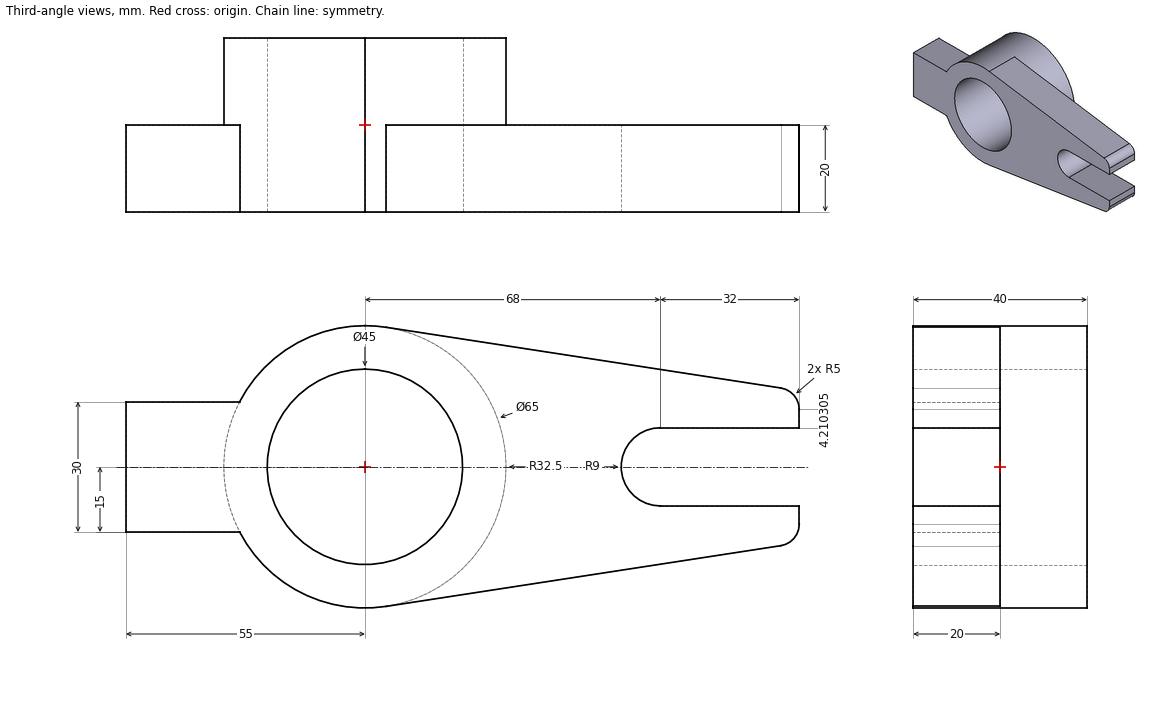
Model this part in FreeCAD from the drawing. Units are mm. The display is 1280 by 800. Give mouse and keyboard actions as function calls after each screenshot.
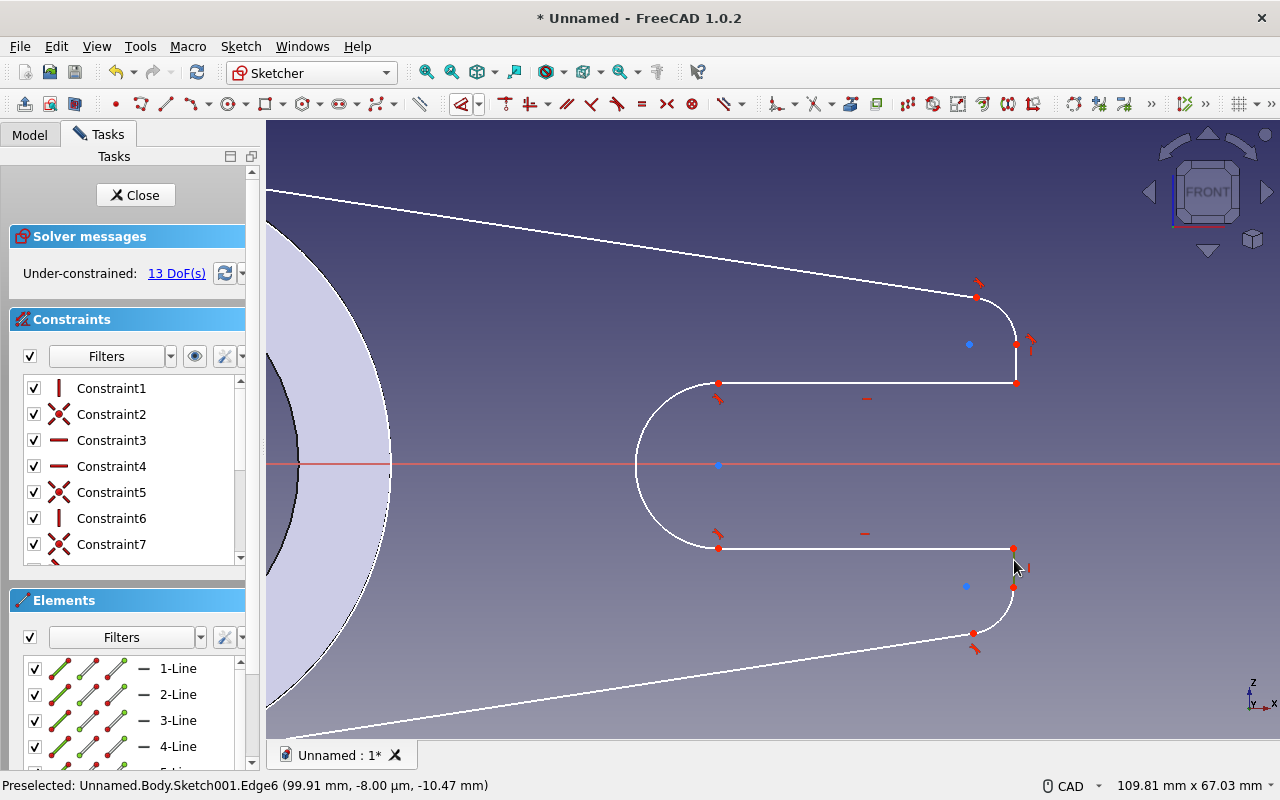
click(992, 627)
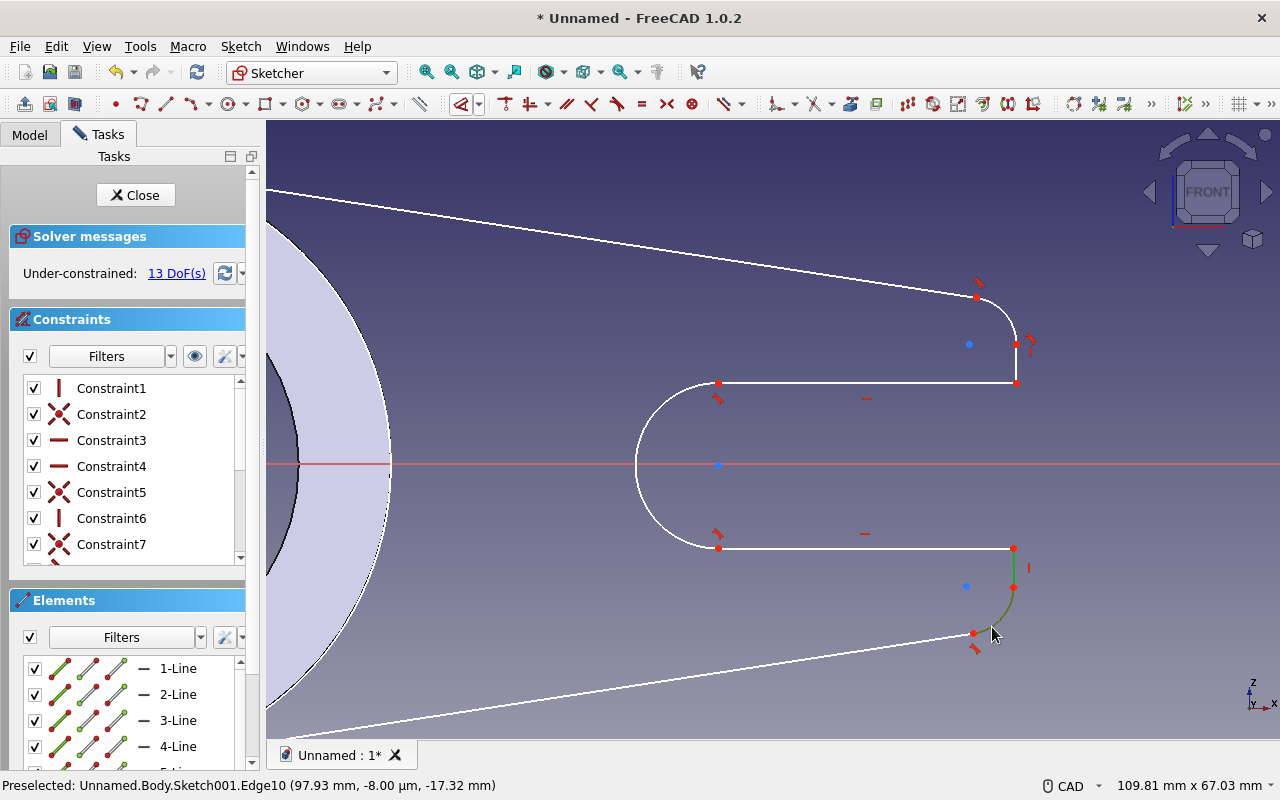
click(617, 104)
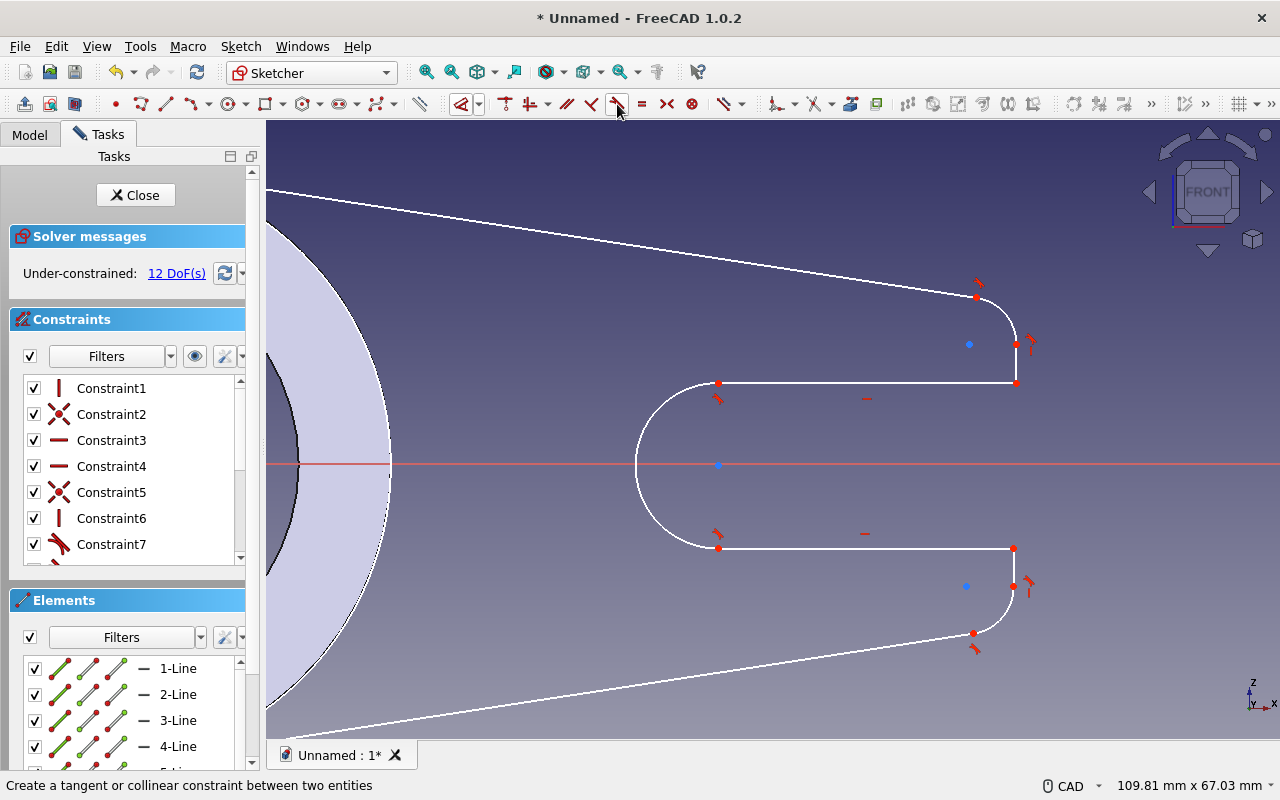
scroll(1013, 359, down, 2)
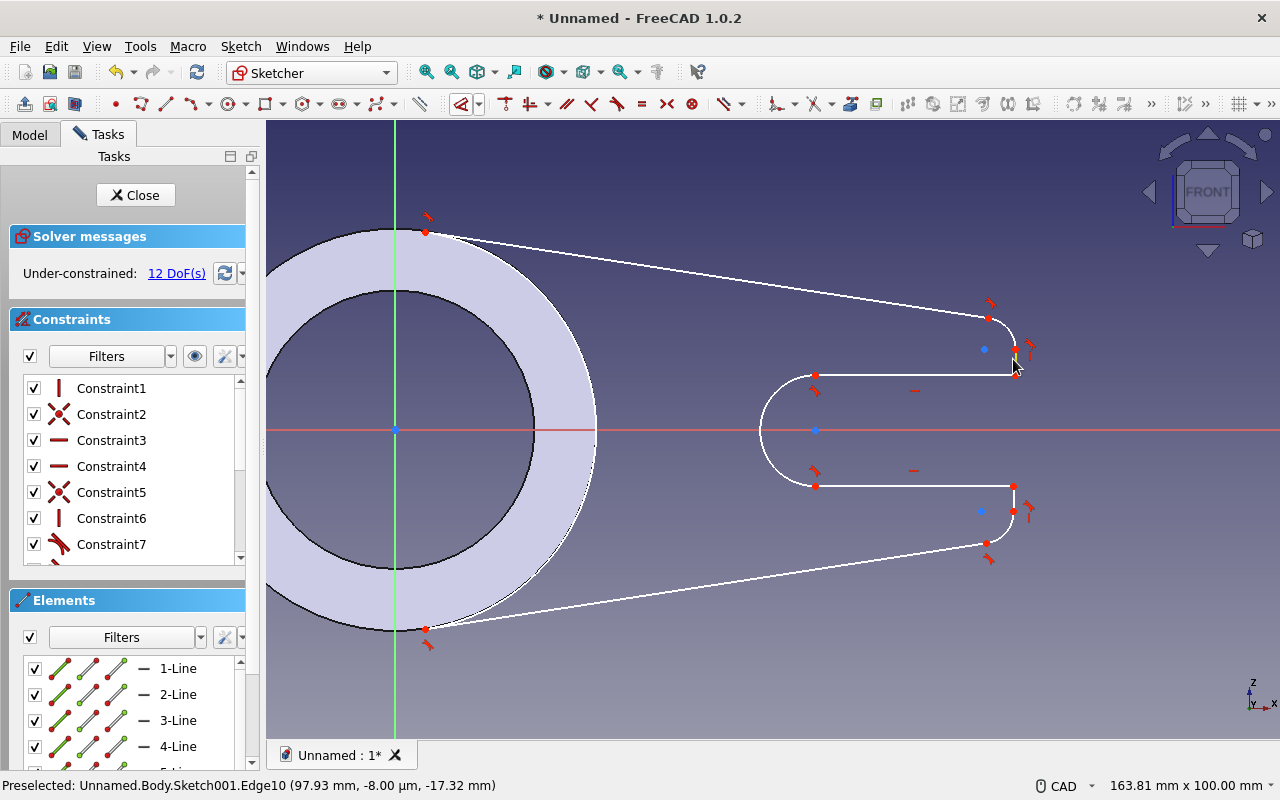
scroll(395, 430, up, 2)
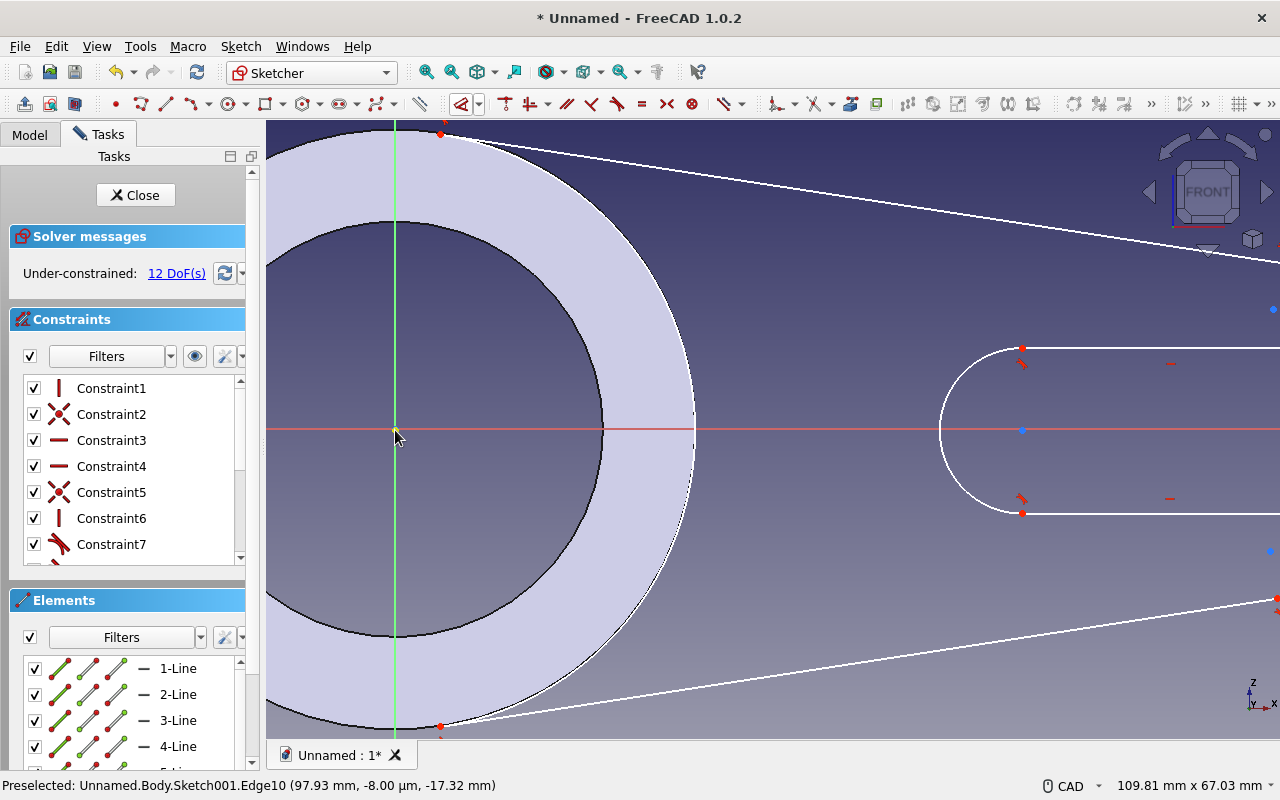
drag(385, 419, 406, 441)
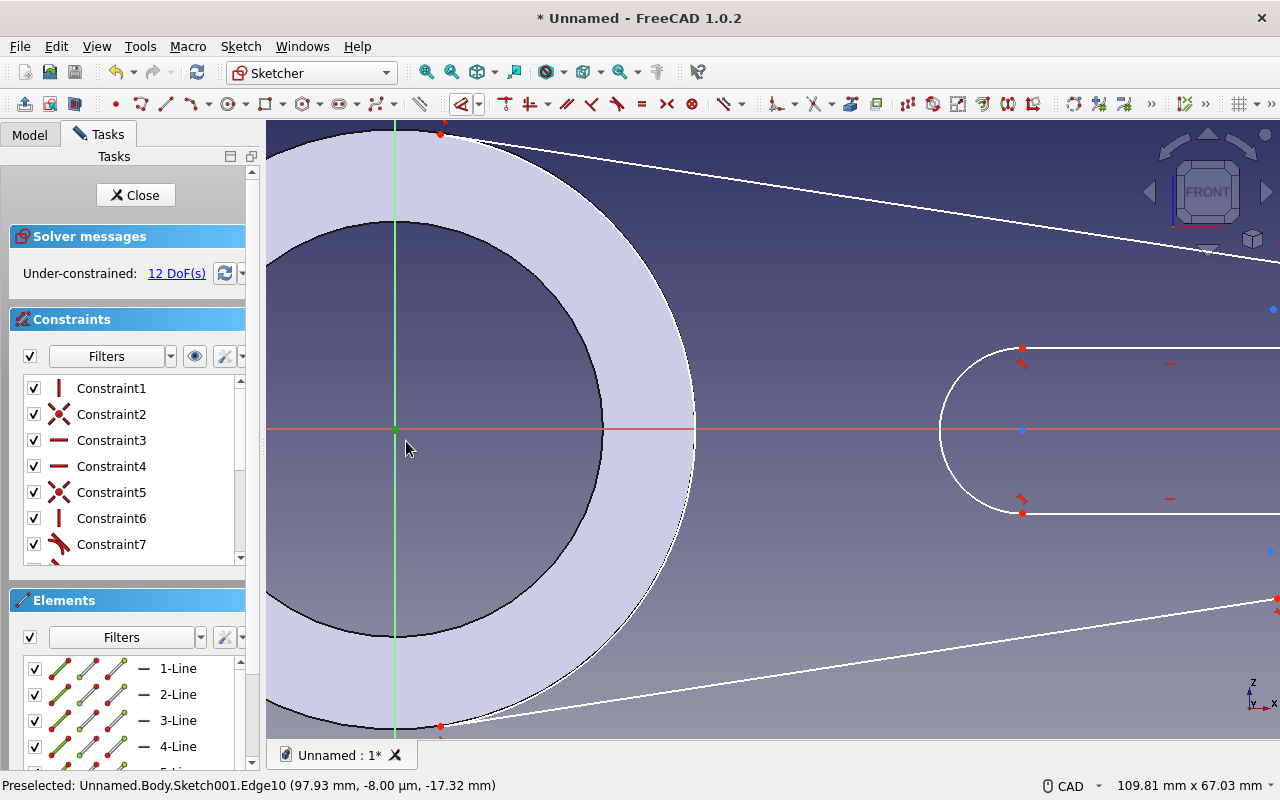
key(c)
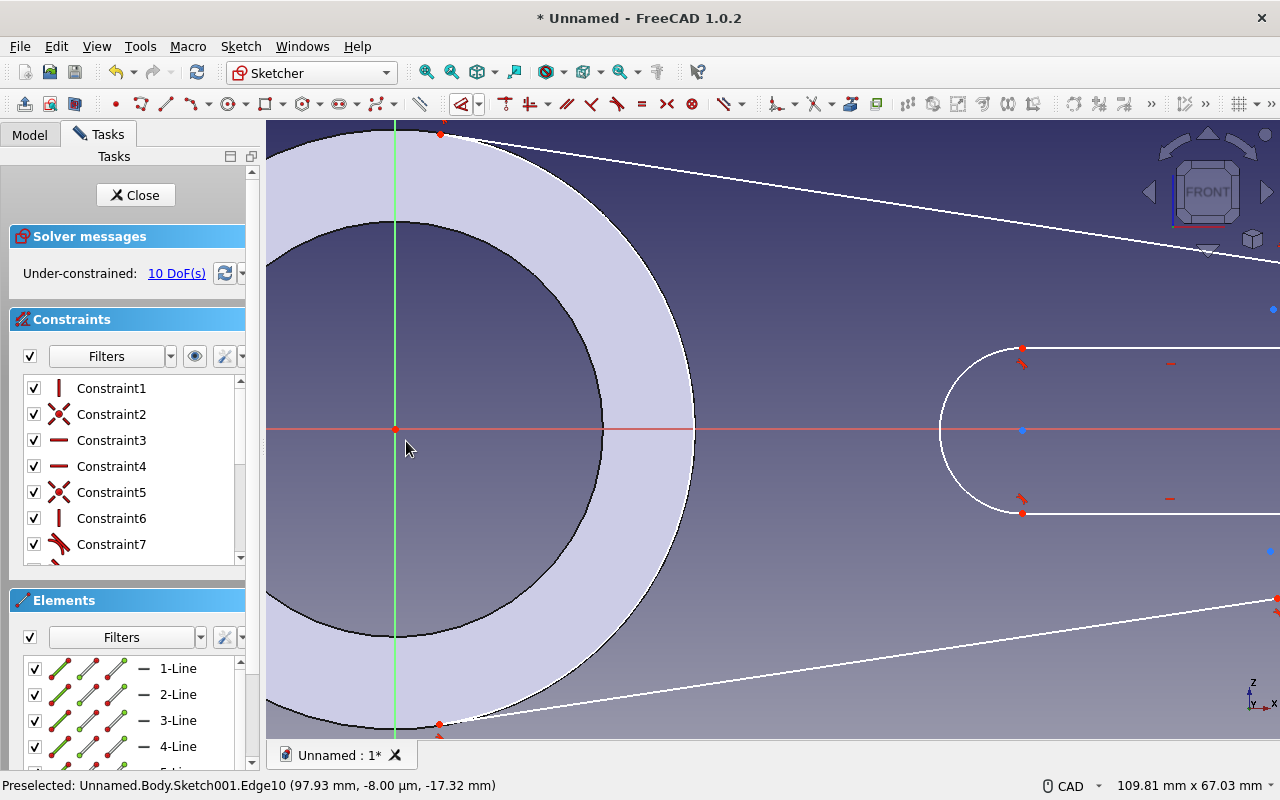
scroll(395, 430, down, 2)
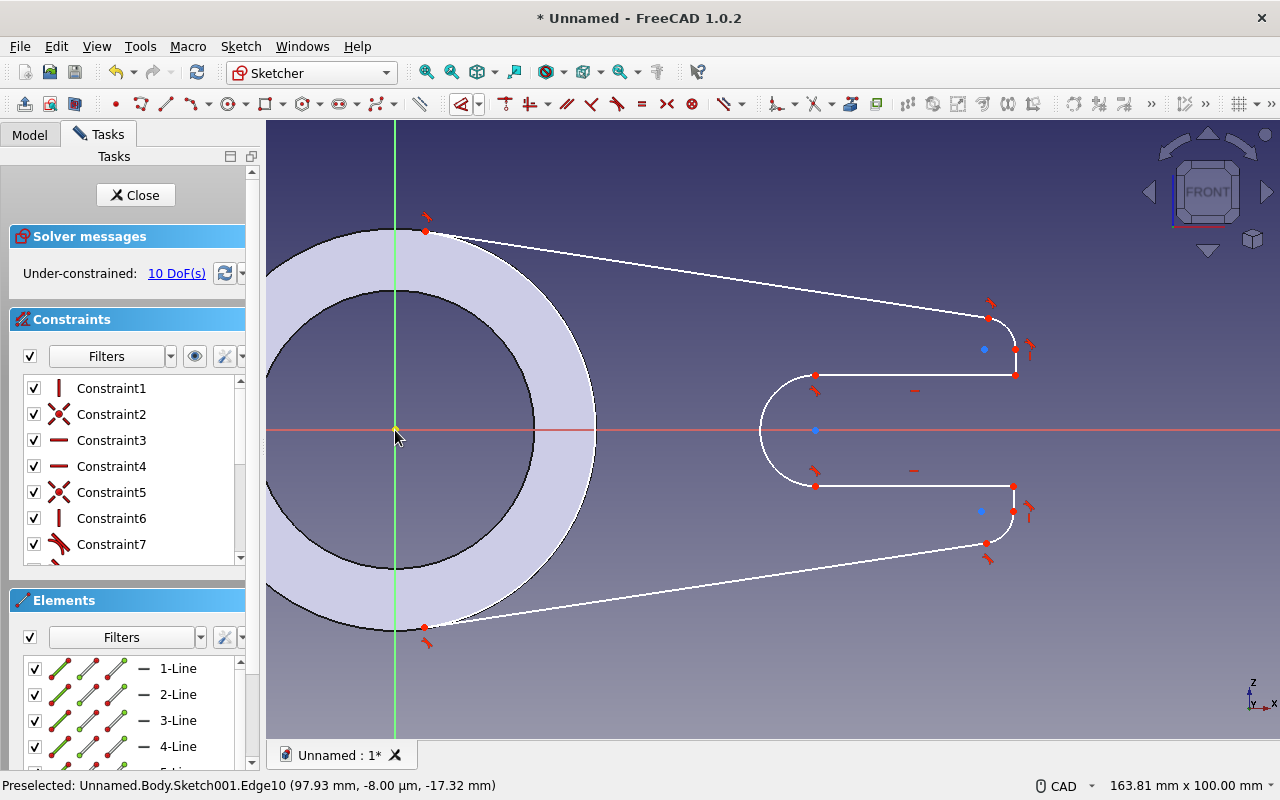
click(1013, 336)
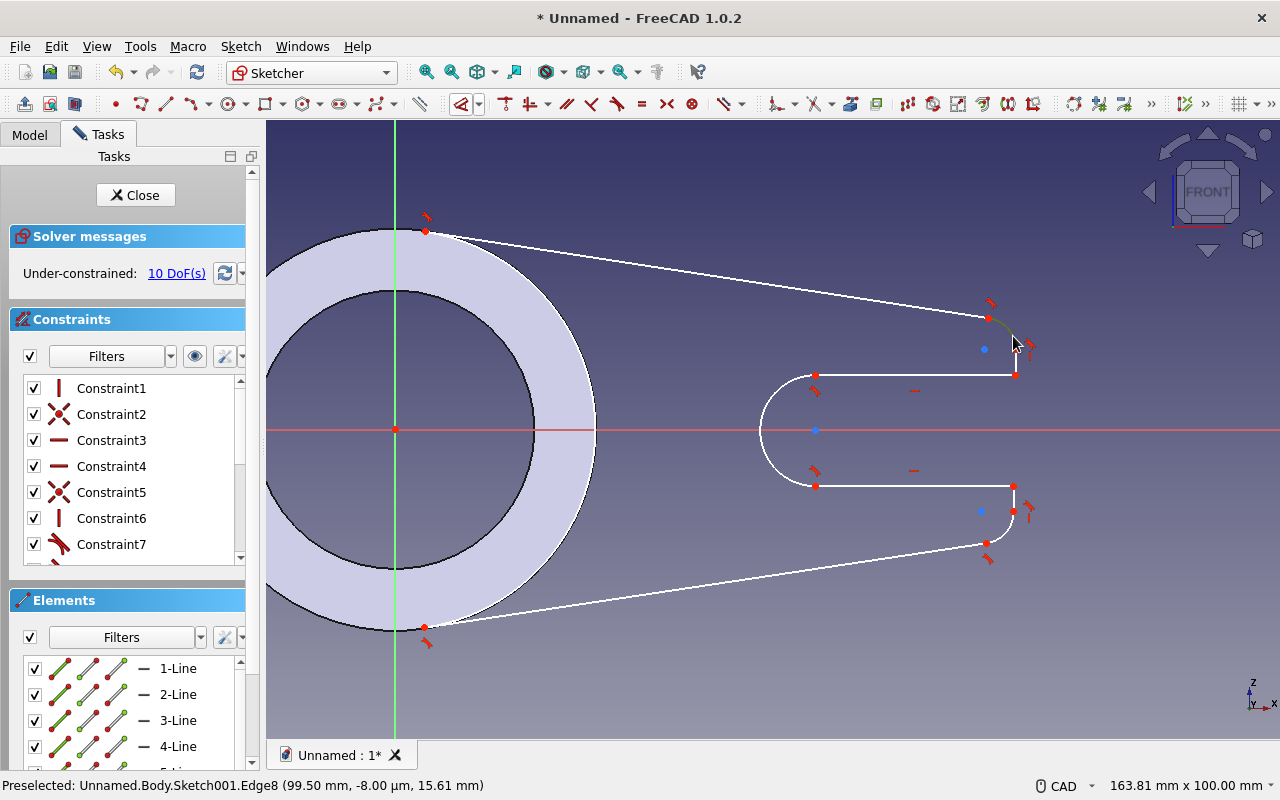
click(999, 538)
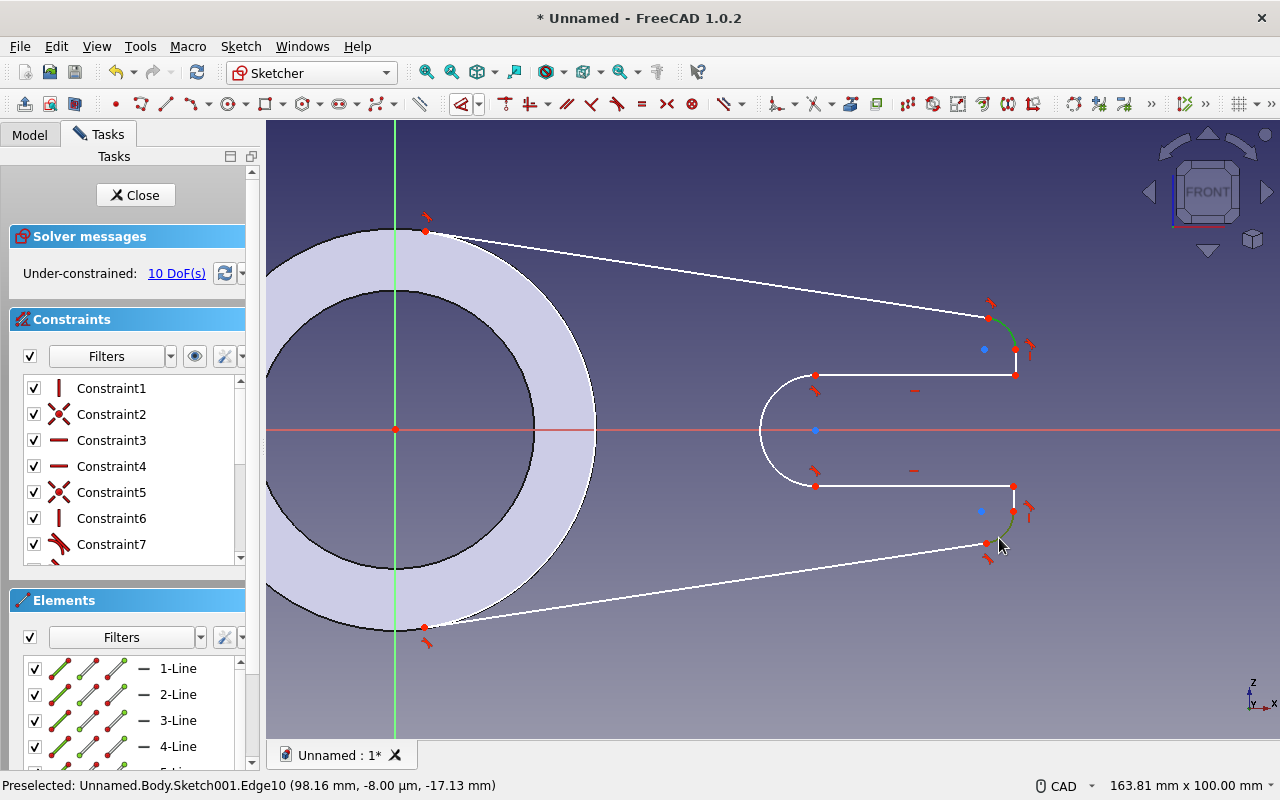
key(e)